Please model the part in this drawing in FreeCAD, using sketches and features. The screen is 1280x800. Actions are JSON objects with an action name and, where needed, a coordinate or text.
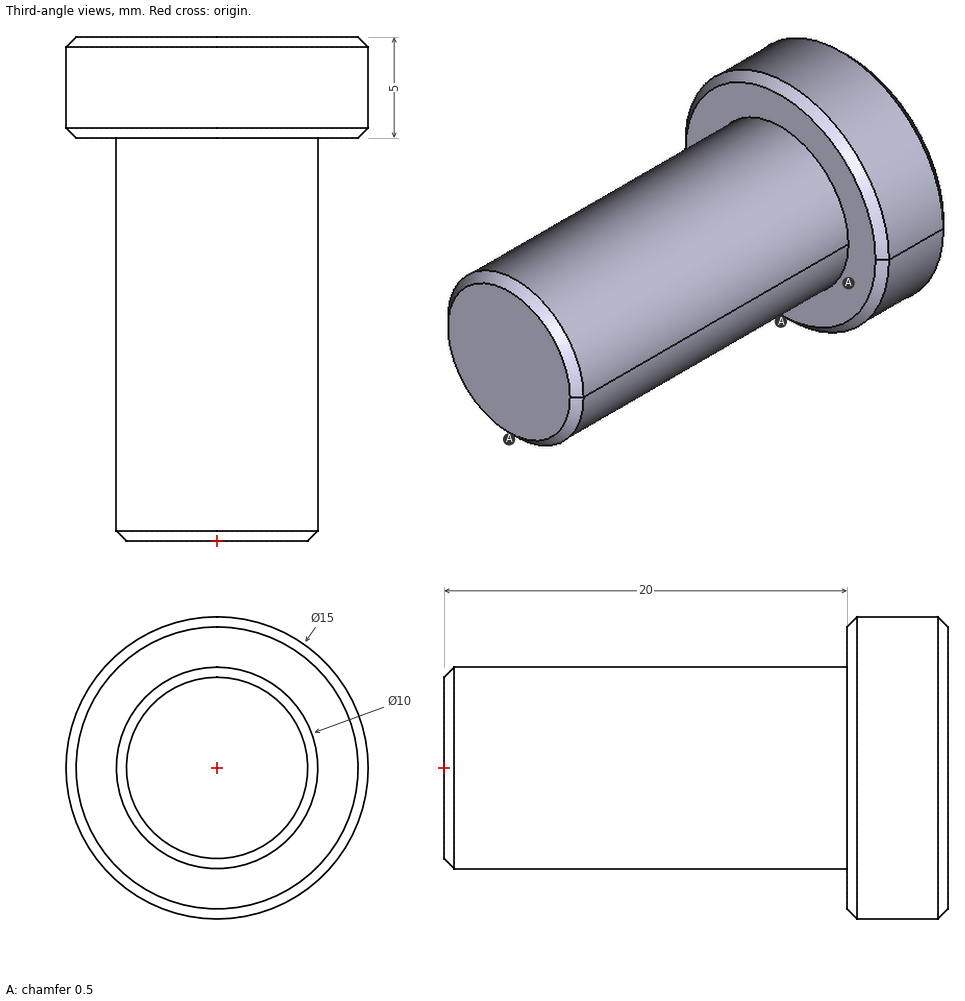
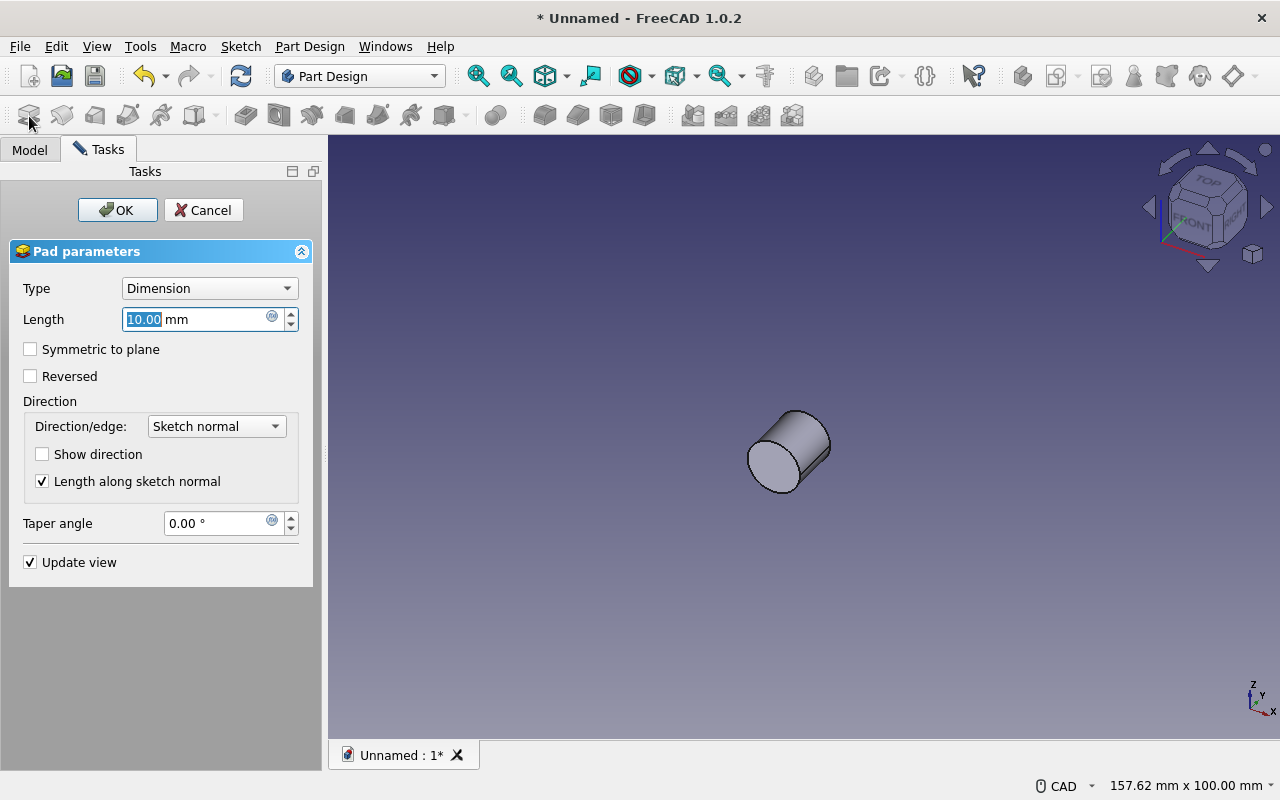
{"action": "type", "text": "20"}
{"action": "key", "text": "Tab"}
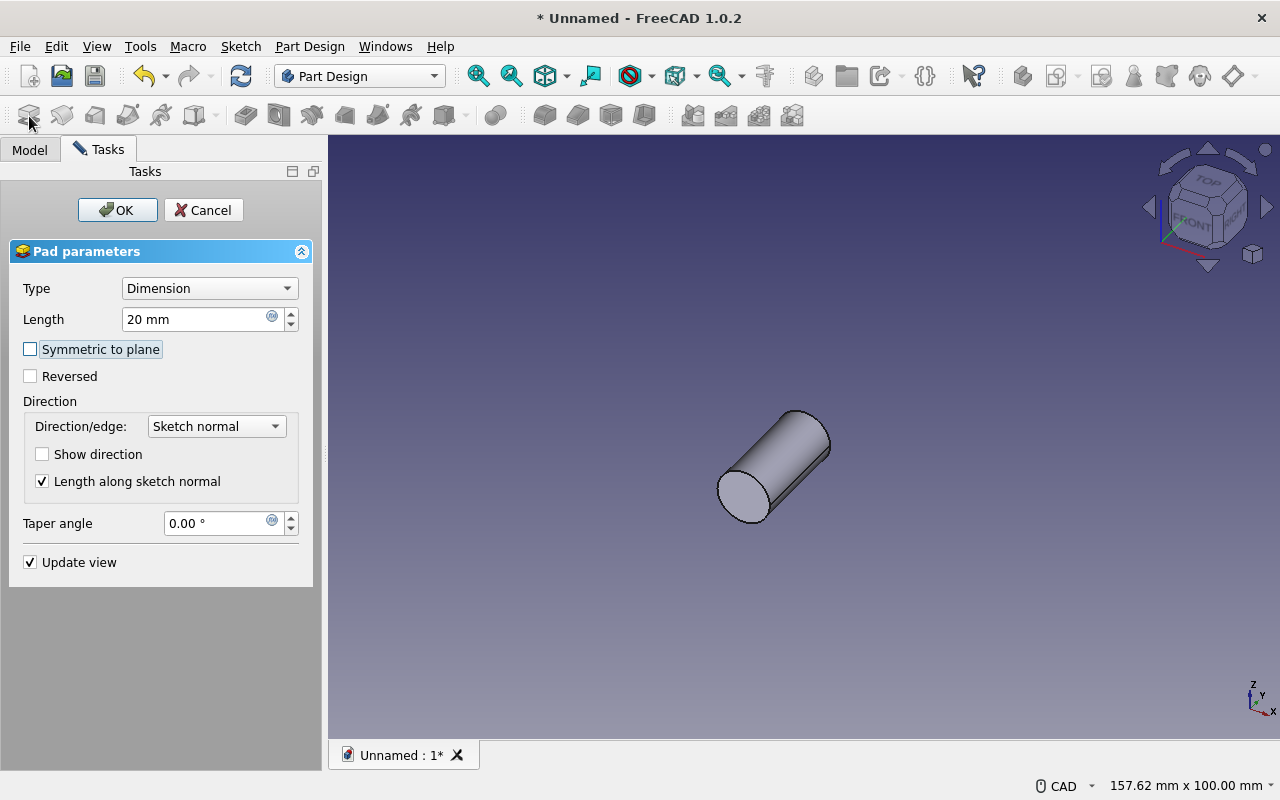
{"action": "left_click", "coordinate": [31, 376]}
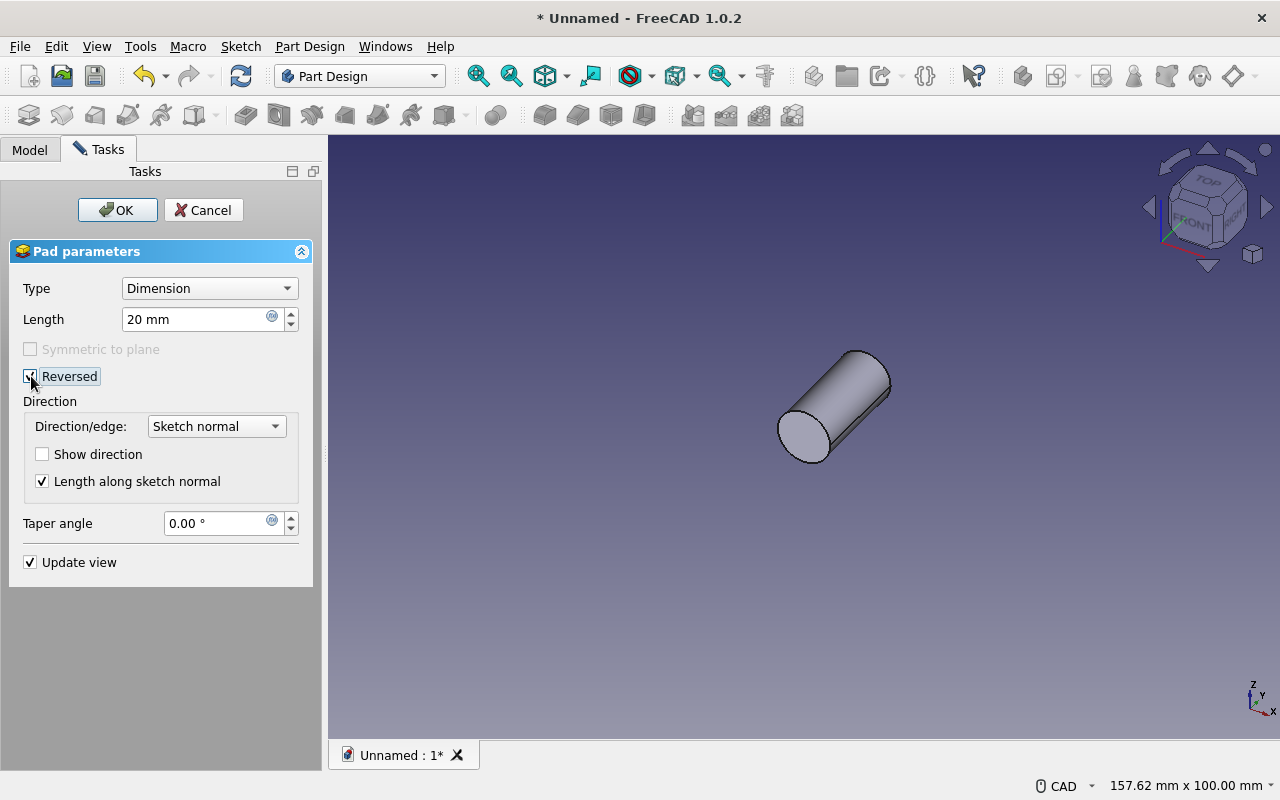
{"action": "left_click", "coordinate": [118, 210]}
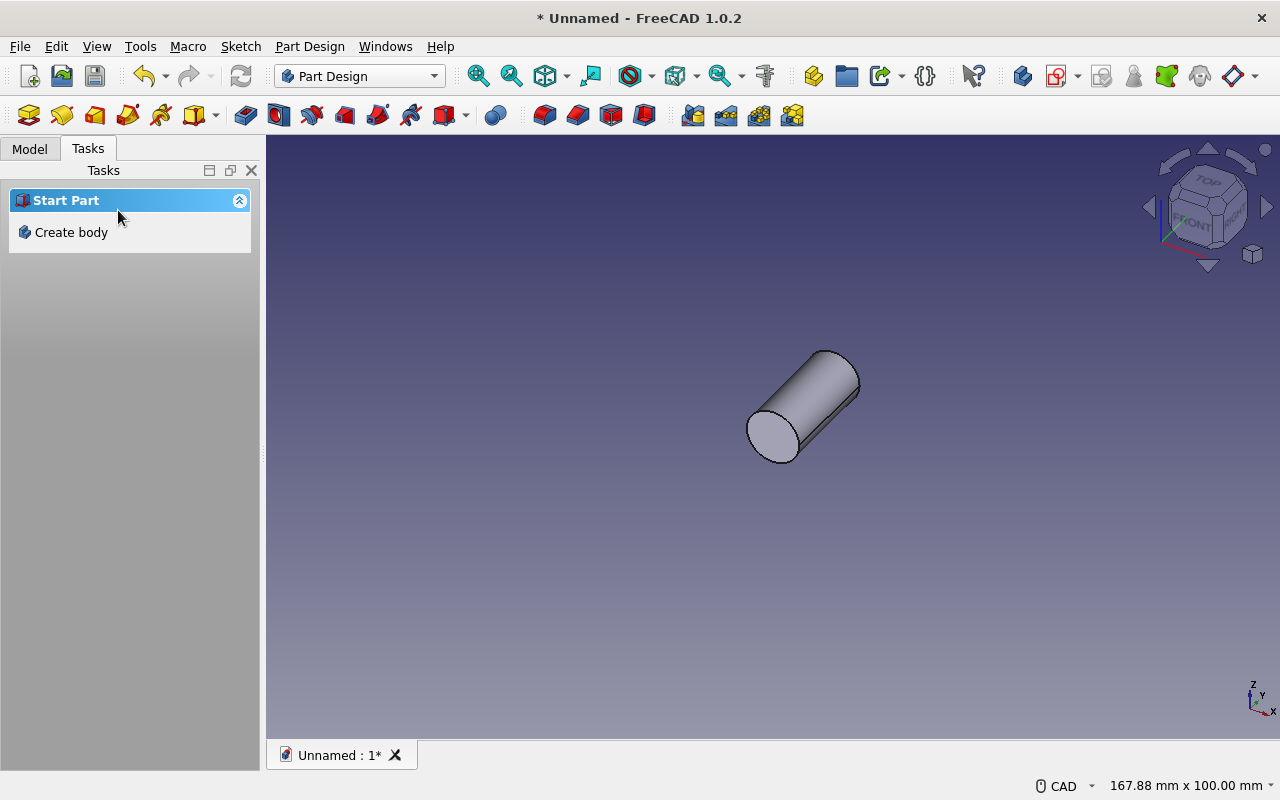
{"action": "left_click", "coordinate": [479, 76]}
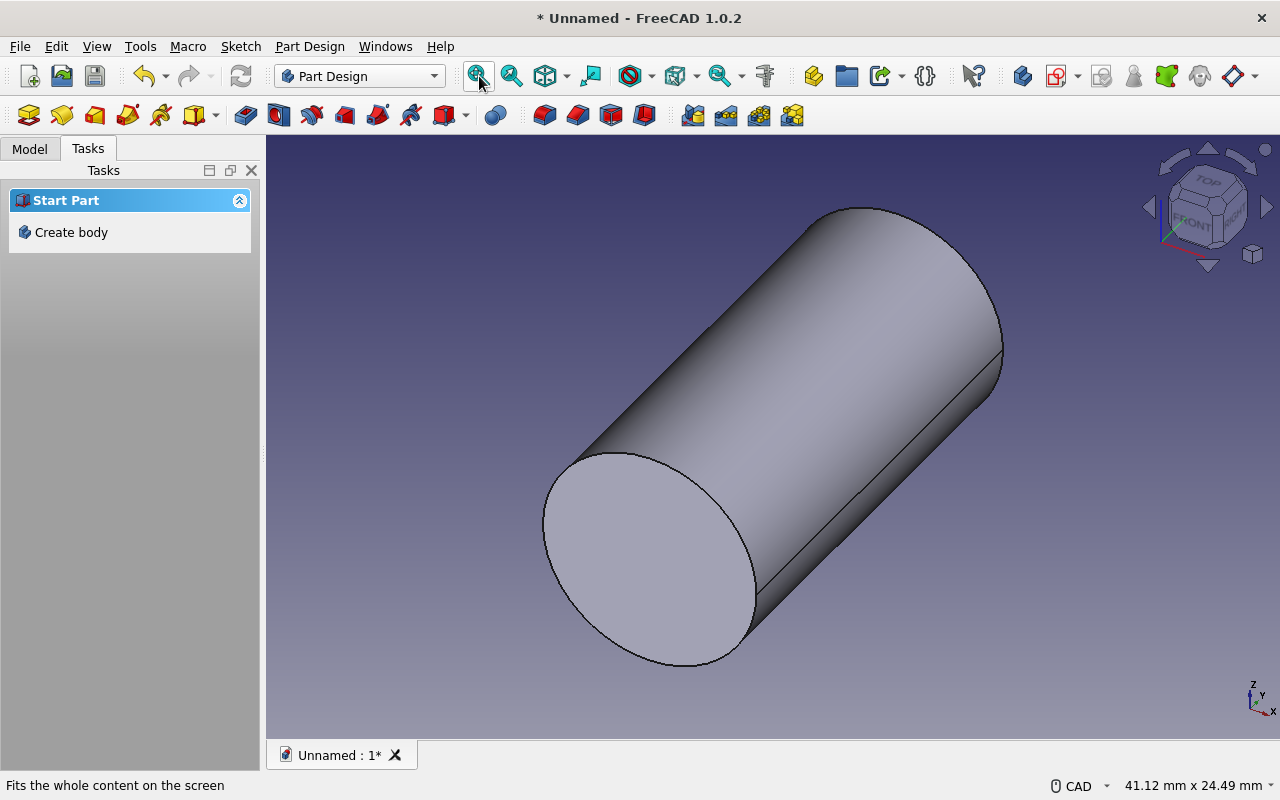
{"action": "key", "text": "4"}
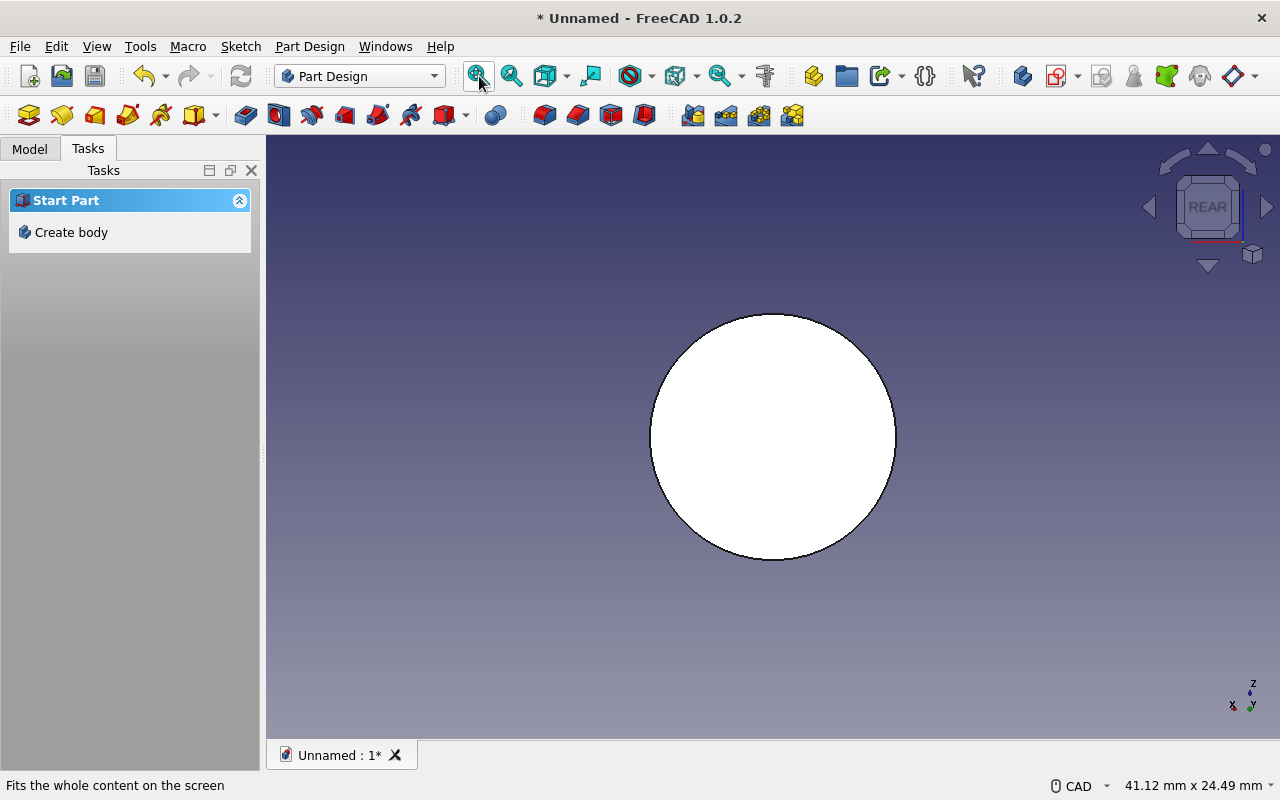
{"action": "key", "text": "v f"}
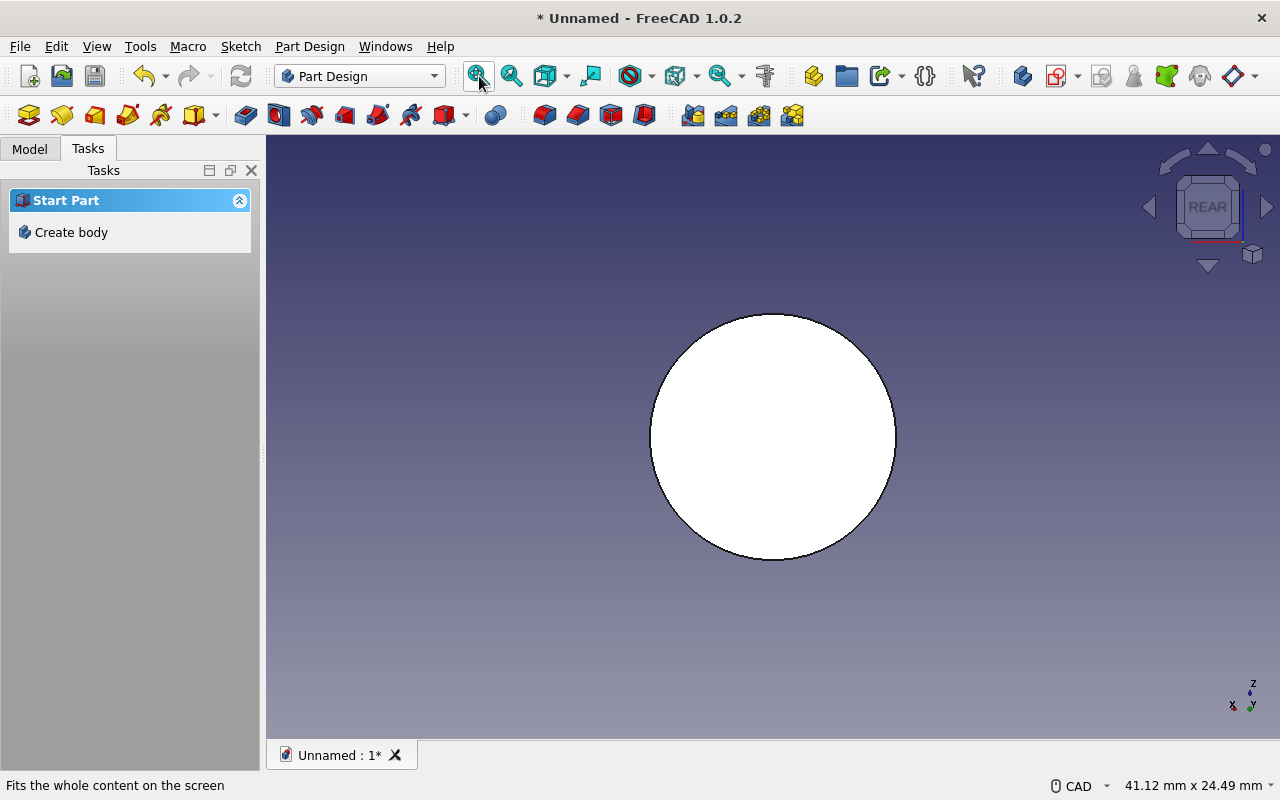
{"action": "left_click", "coordinate": [773, 436]}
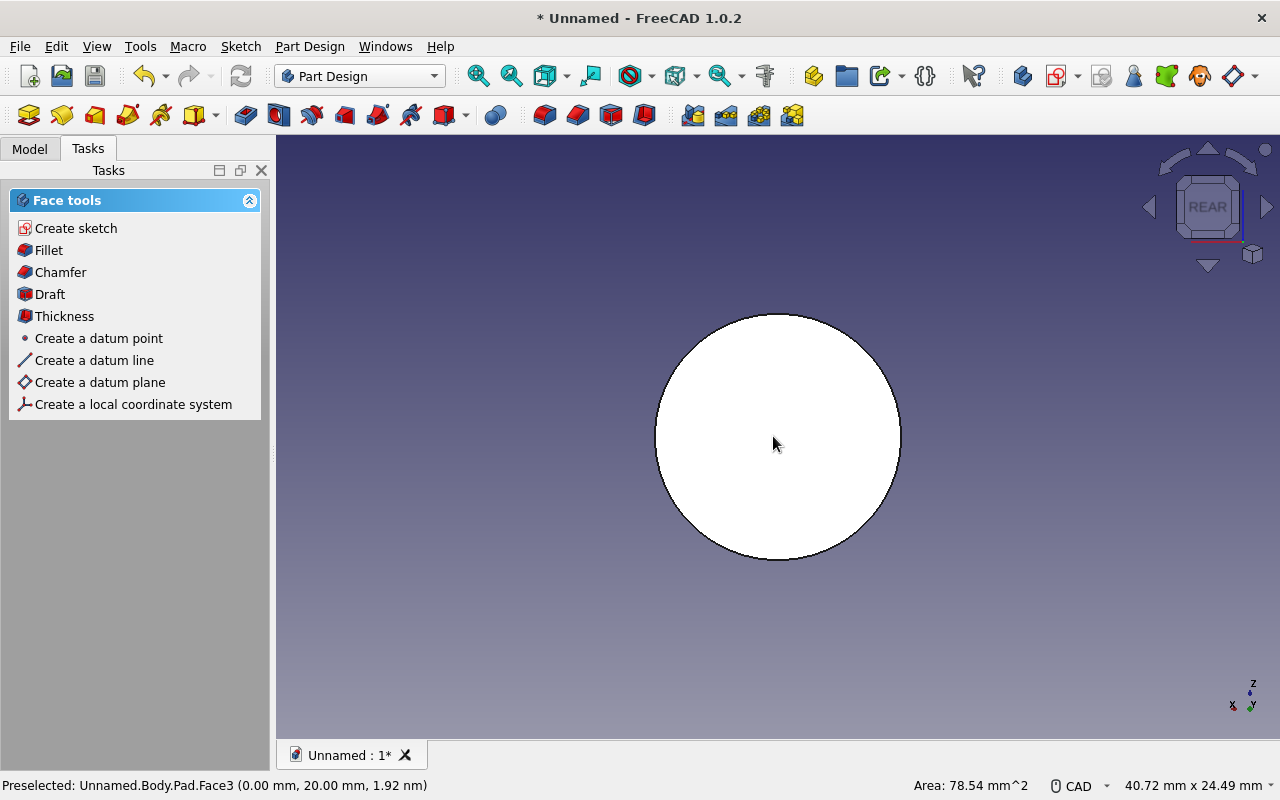
{"action": "left_click", "coordinate": [1056, 76]}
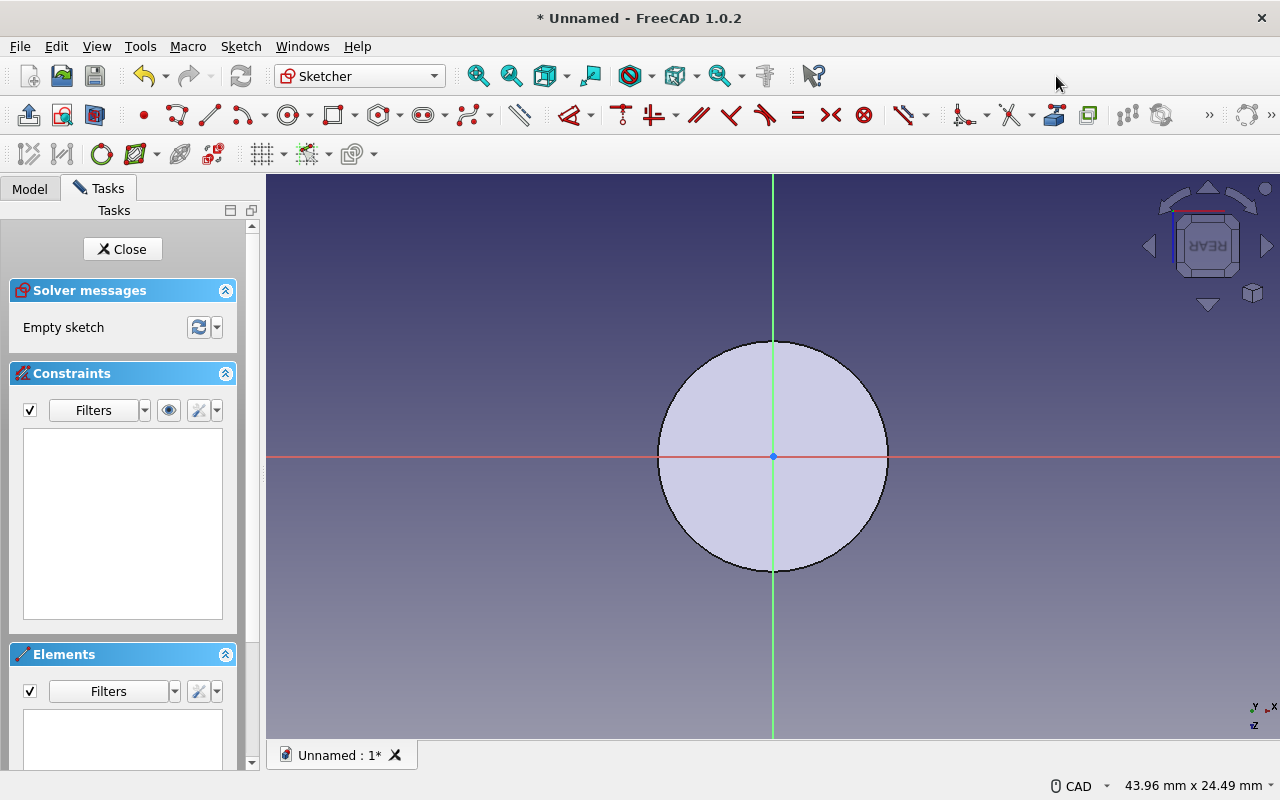
{"action": "key", "text": "g c"}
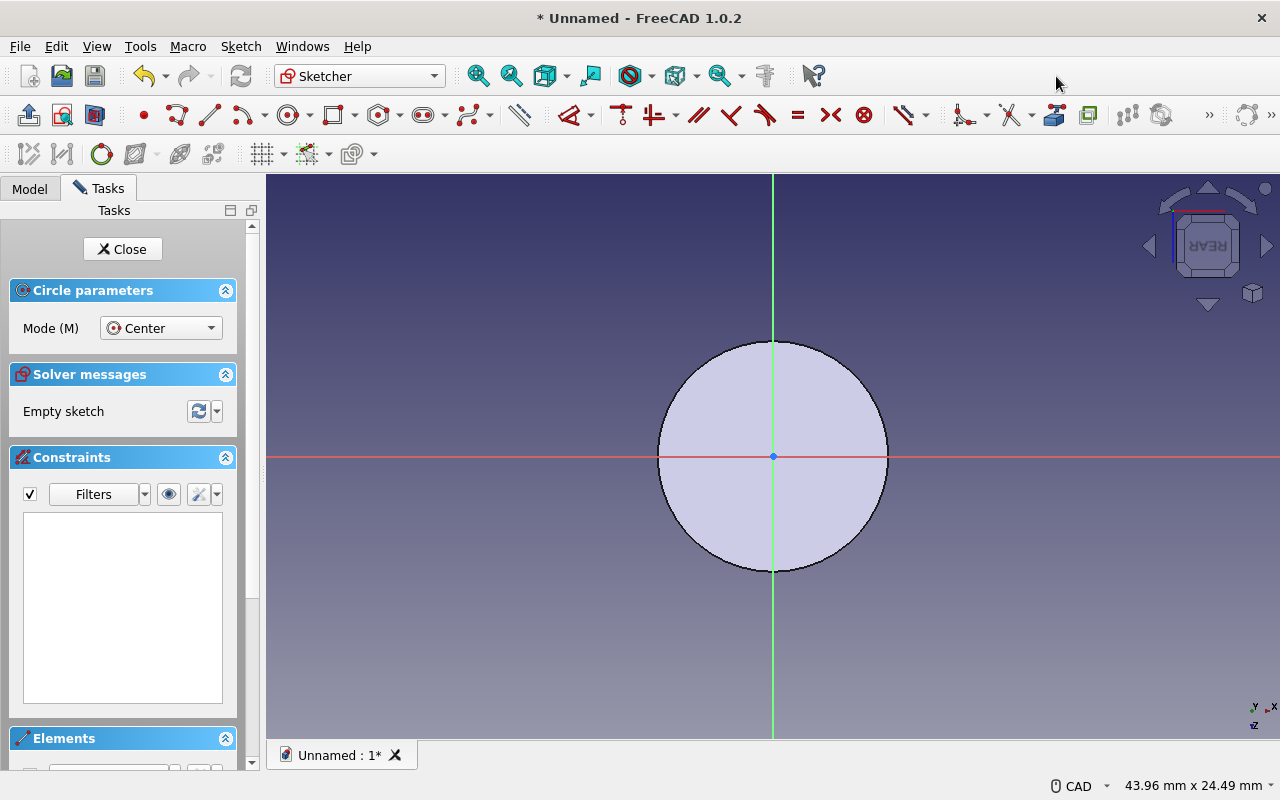
{"action": "left_click", "coordinate": [773, 456]}
{"action": "mouse_move", "coordinate": [895, 334]}